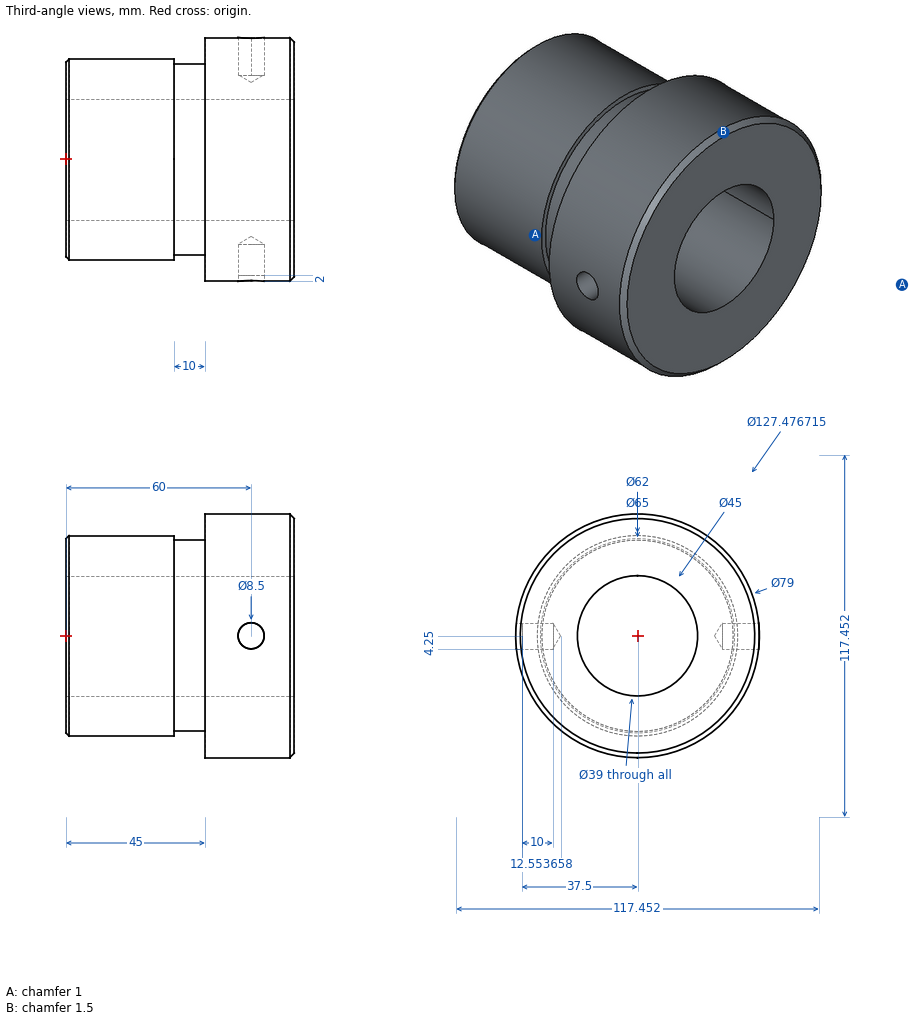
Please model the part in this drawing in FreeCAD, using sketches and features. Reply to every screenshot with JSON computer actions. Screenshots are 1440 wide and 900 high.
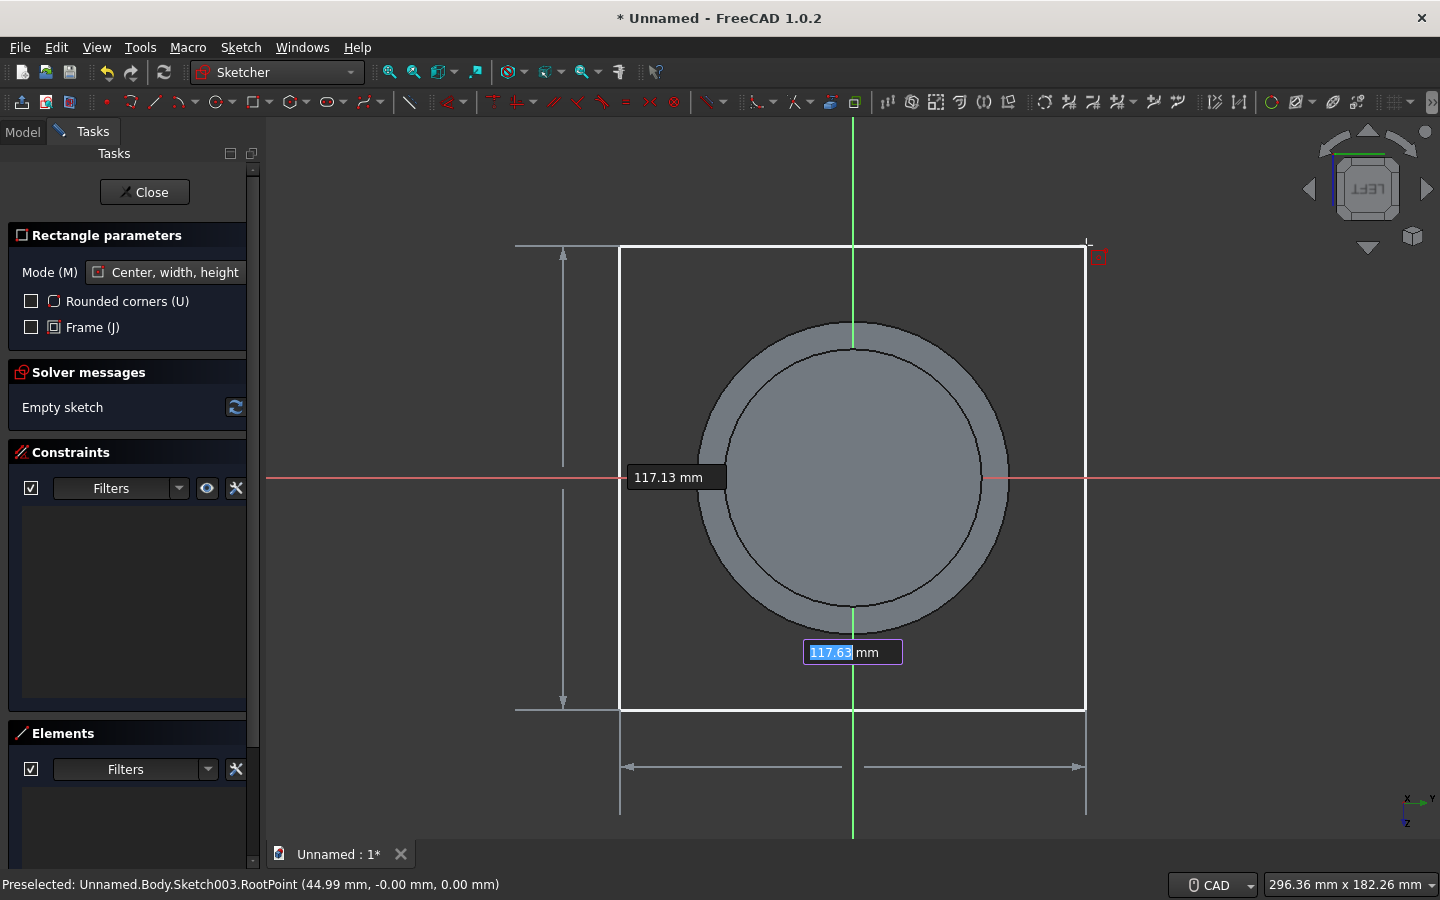
{"action": "type", "text": "117.452"}
{"action": "key", "text": "Tab"}
{"action": "type", "text": "117.452"}
{"action": "key", "text": "Return"}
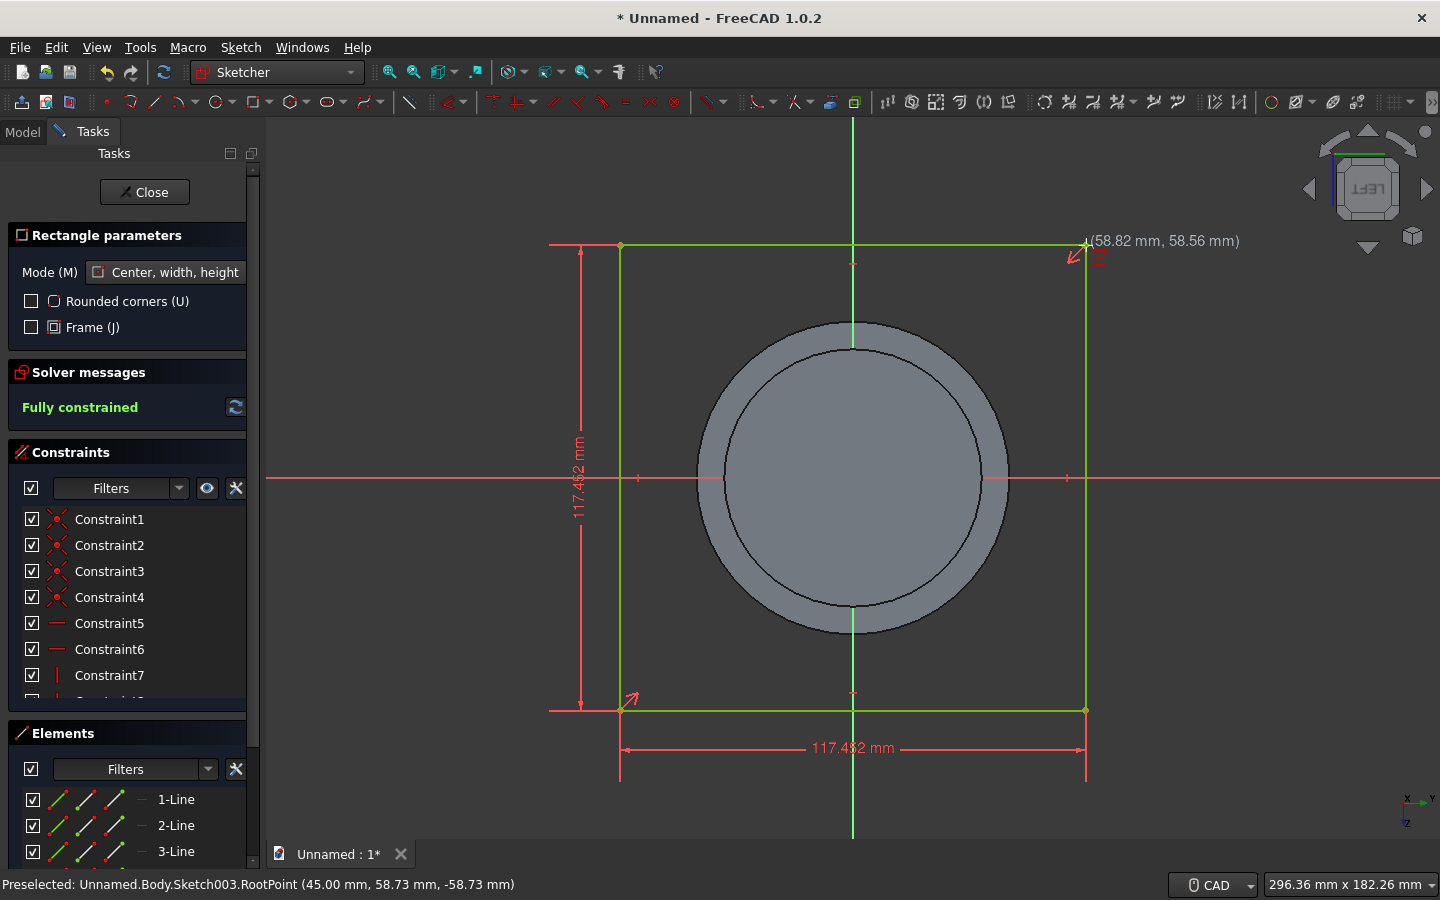
{"action": "key", "text": "g c"}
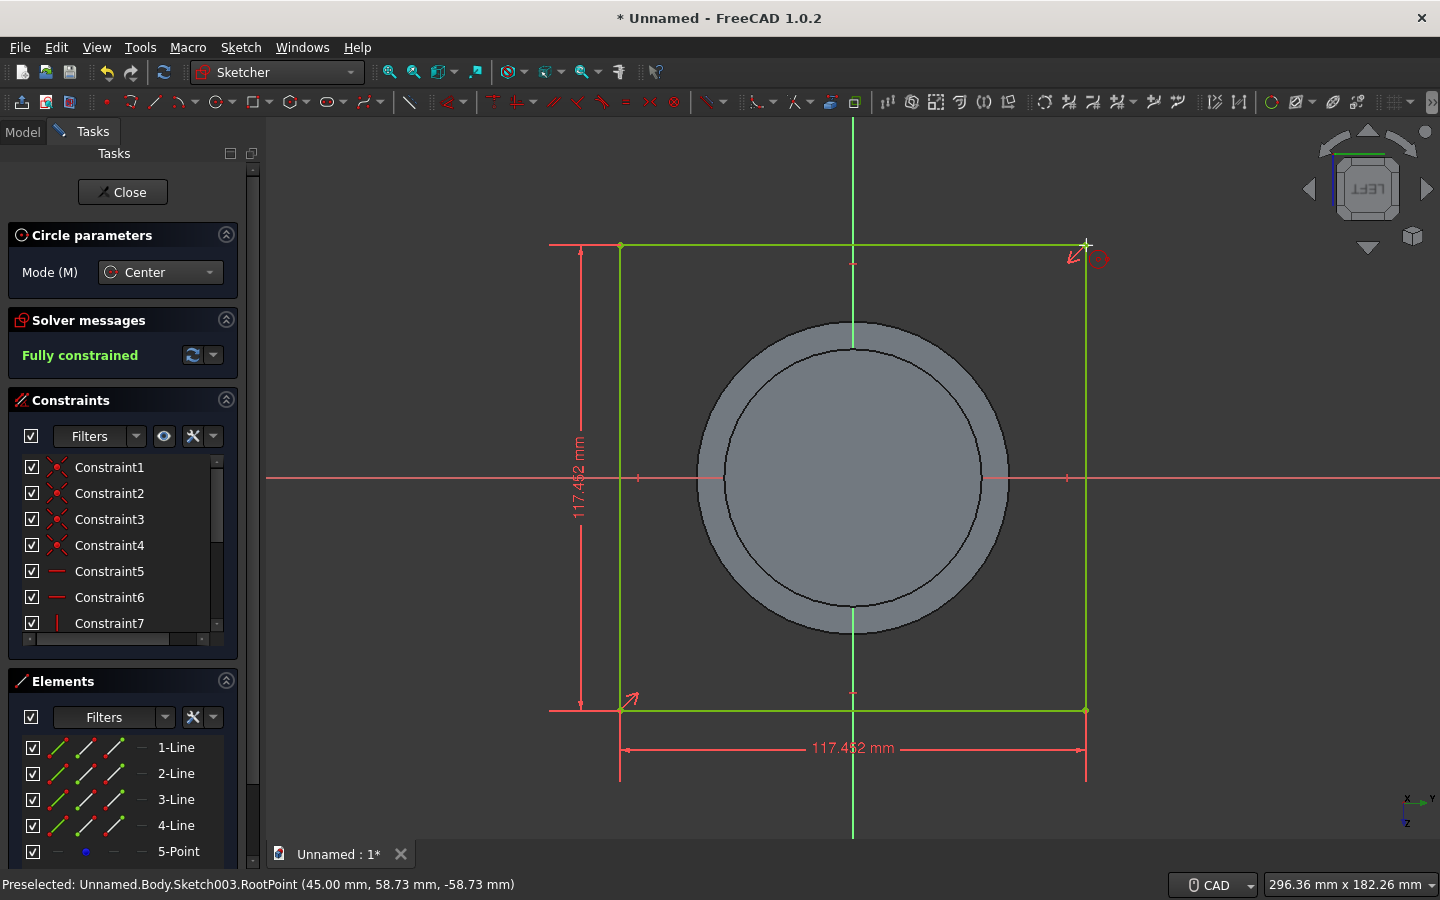
{"action": "left_click", "coordinate": [853, 478]}
{"action": "mouse_move", "coordinate": [940, 391]}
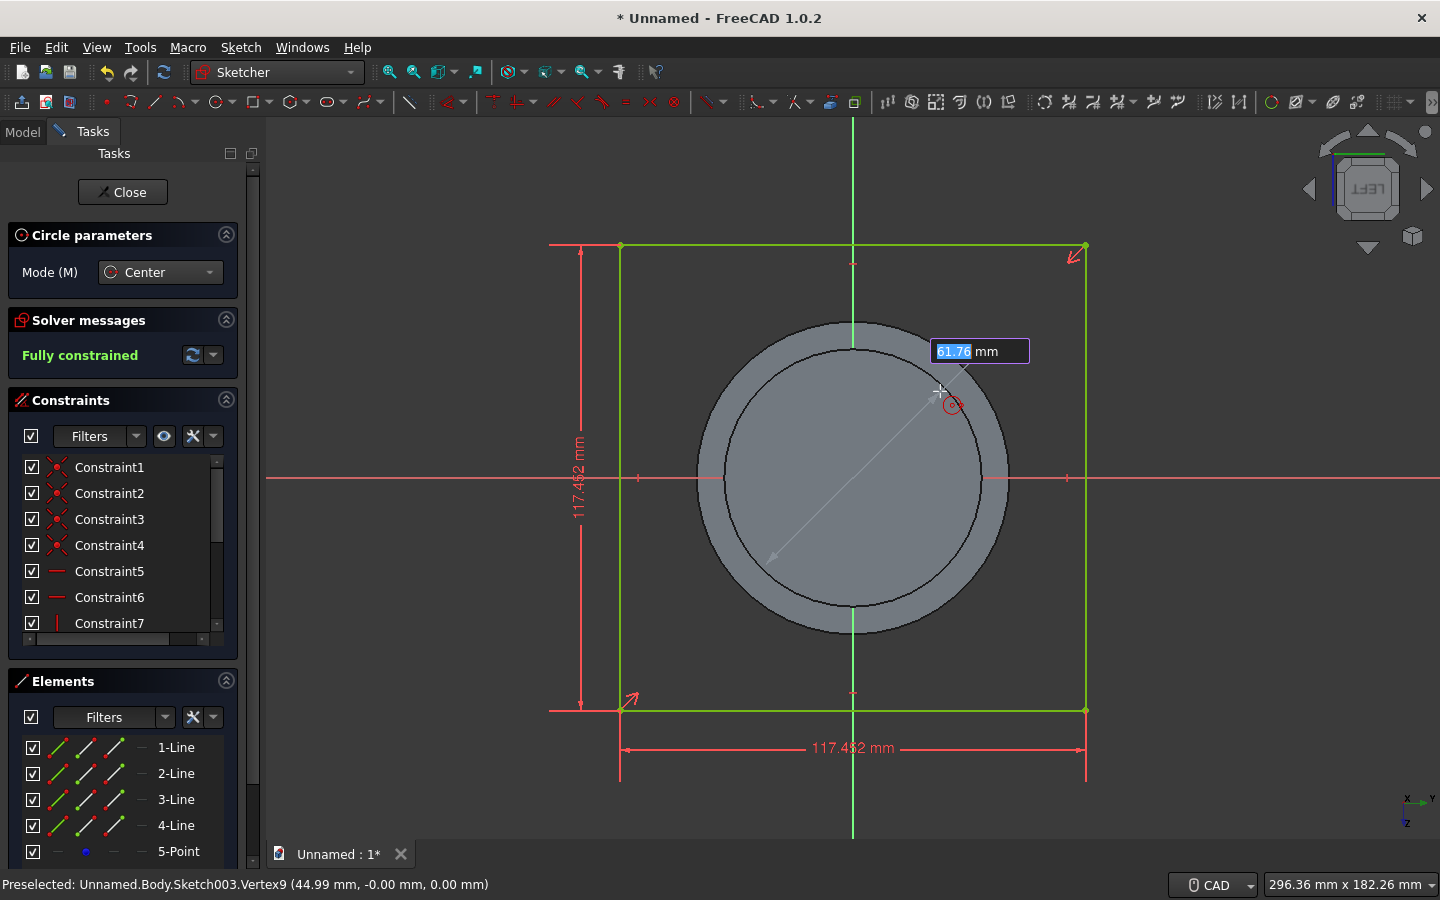
{"action": "type", "text": "62"}
{"action": "key", "text": "Return"}
{"action": "key", "text": "Escape"}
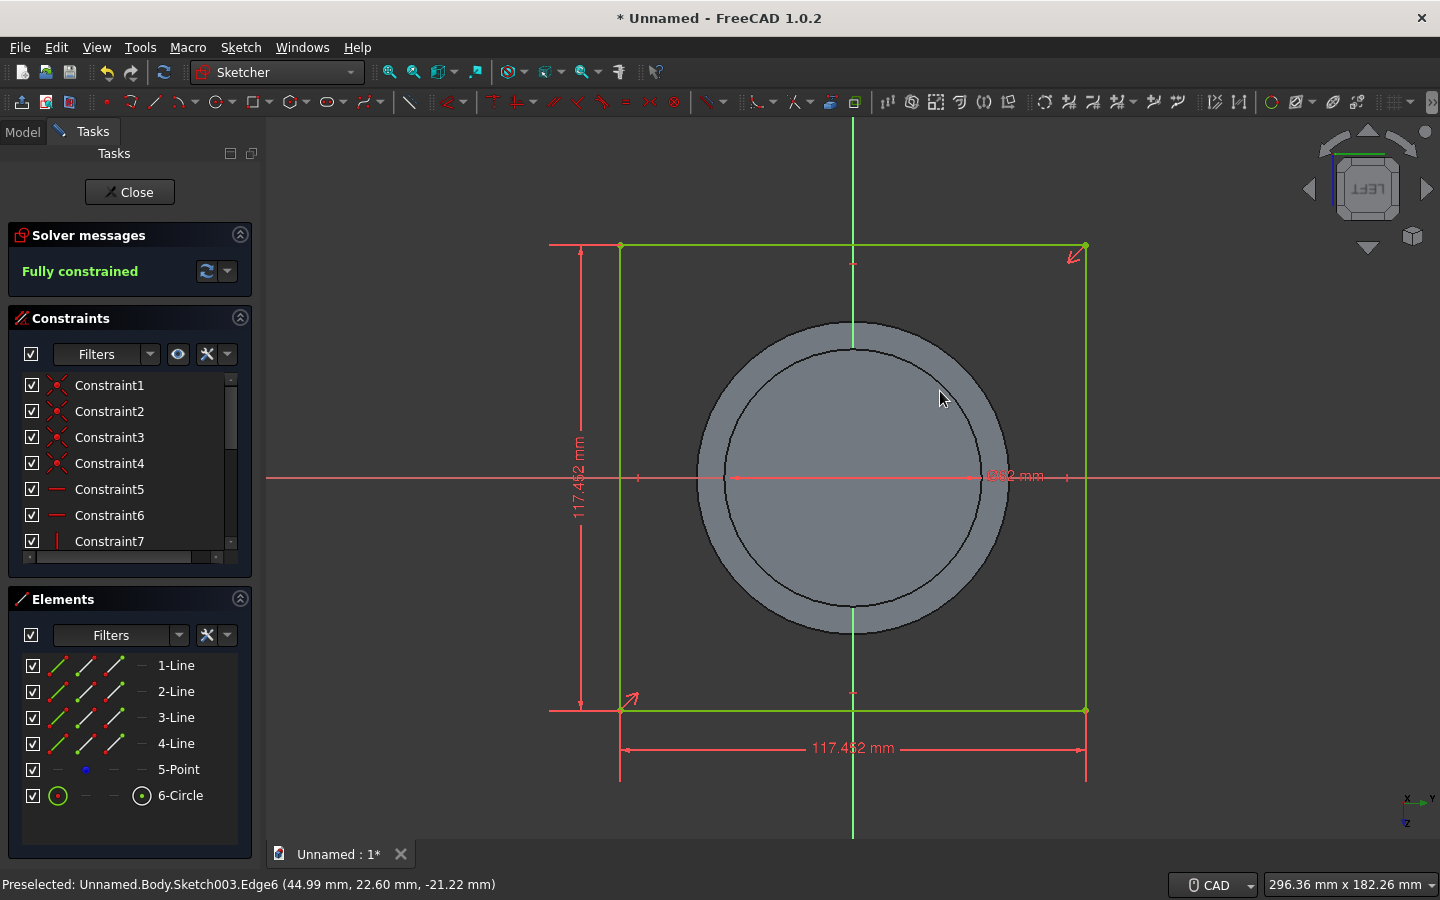
{"action": "left_click", "coordinate": [130, 192]}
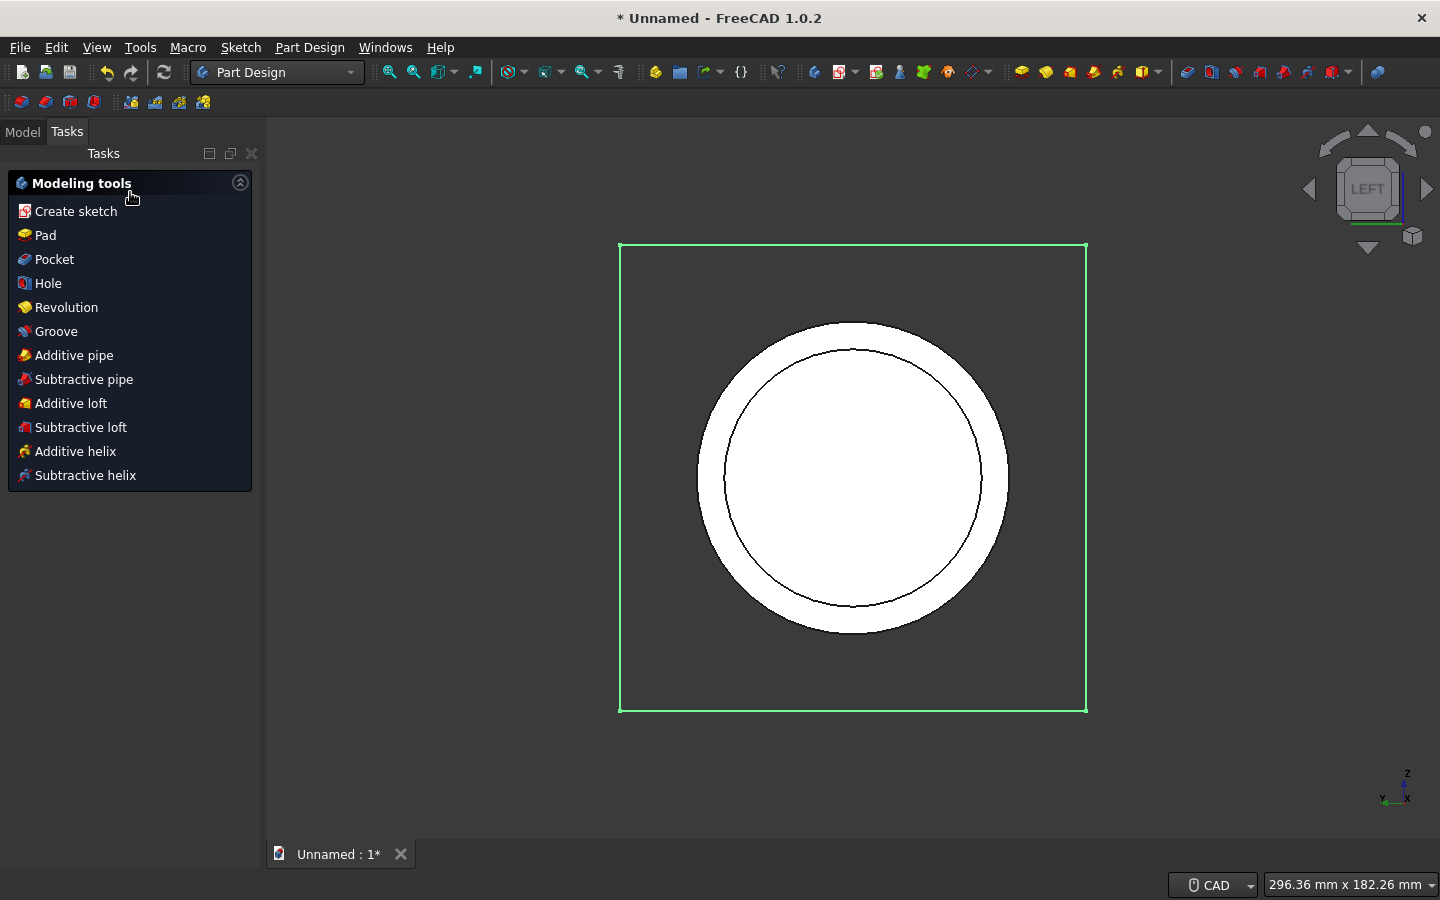
{"action": "left_click", "coordinate": [1188, 72]}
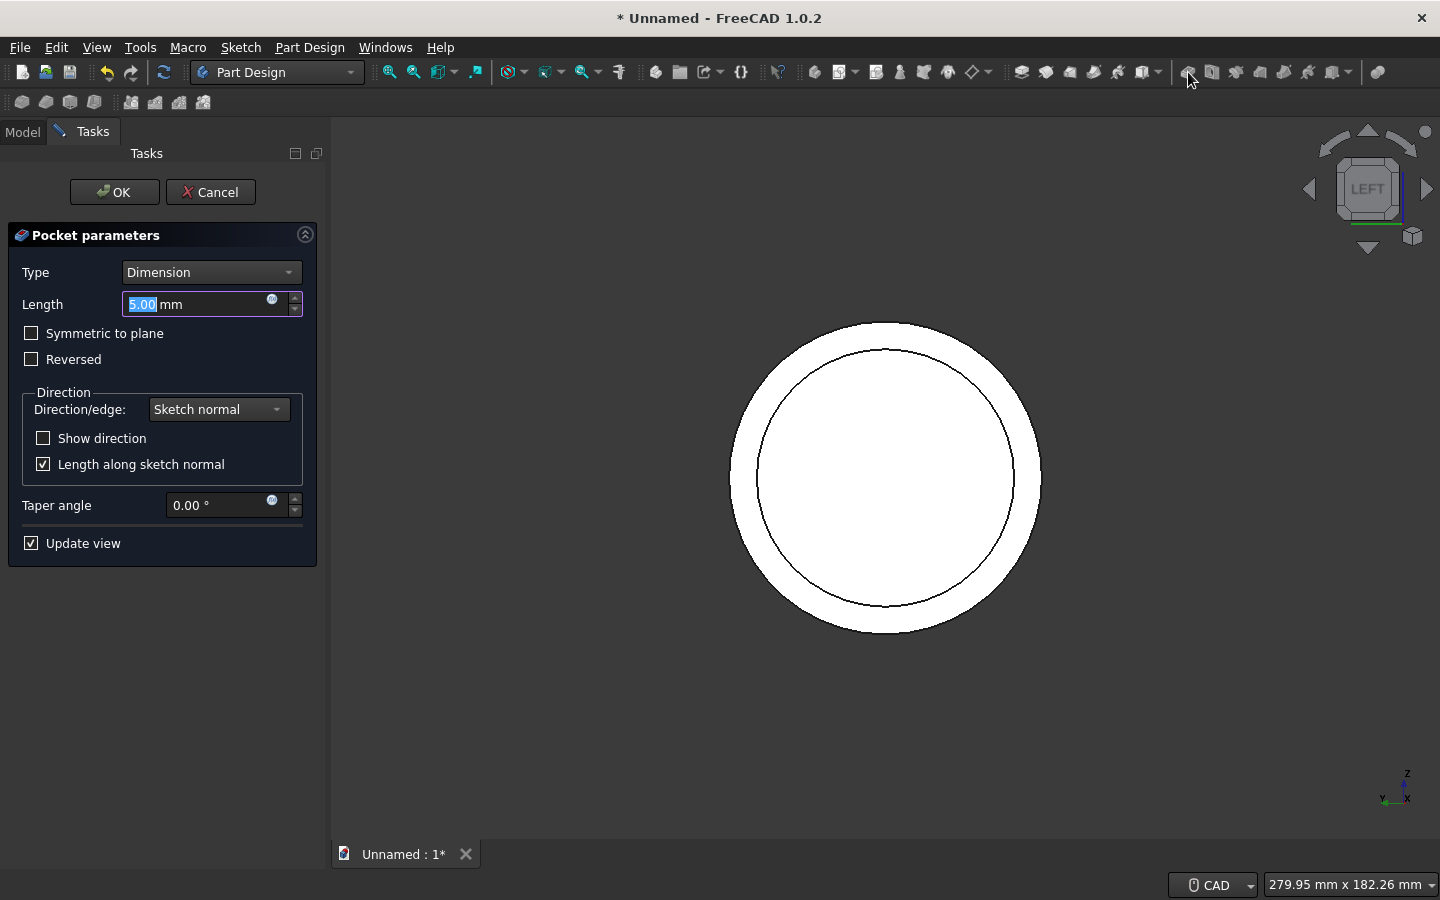
{"action": "type", "text": "10"}
{"action": "key", "text": "Tab"}